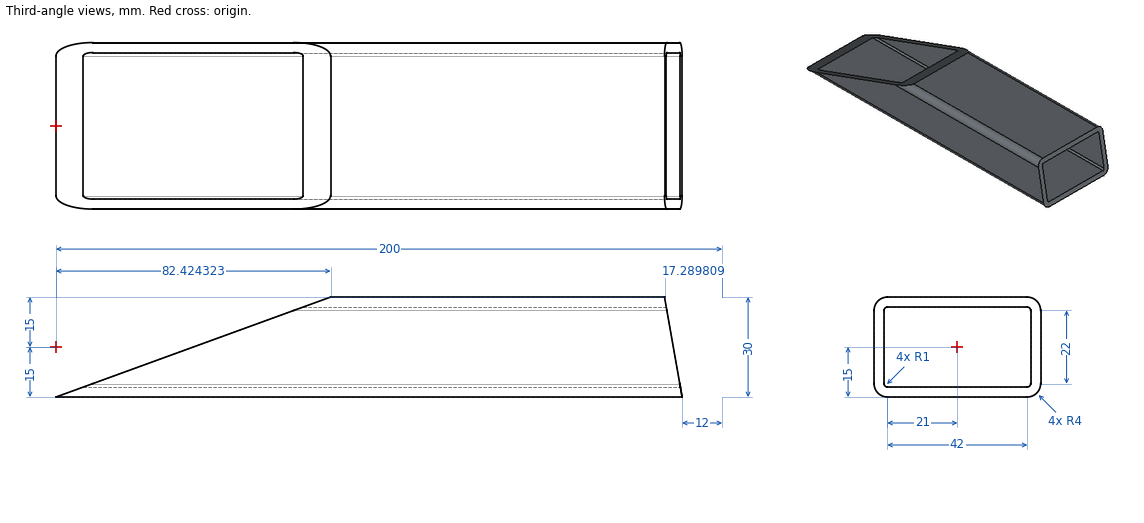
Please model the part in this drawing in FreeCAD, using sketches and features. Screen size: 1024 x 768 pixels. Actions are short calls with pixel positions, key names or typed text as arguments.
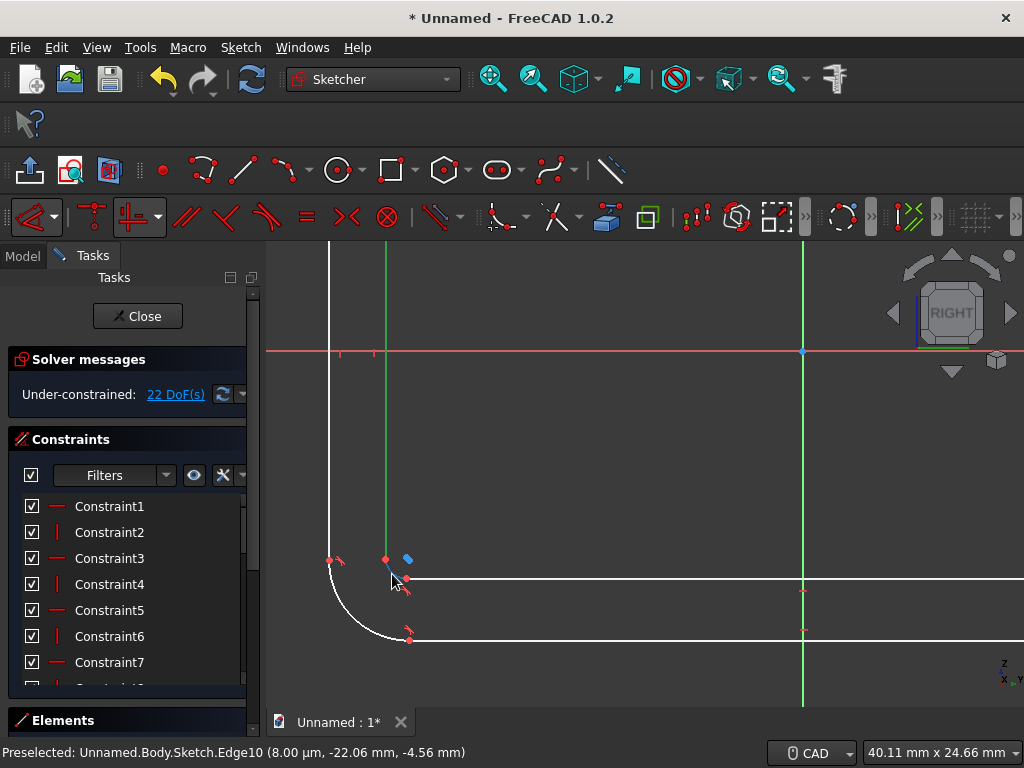
click(393, 573)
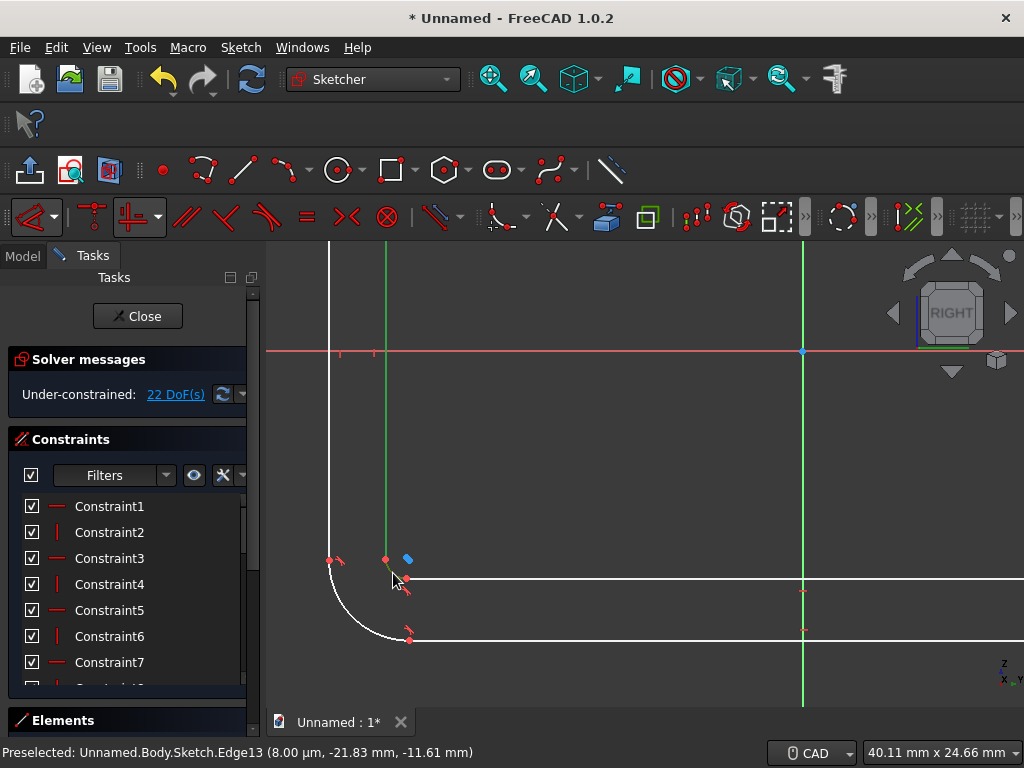
click(268, 218)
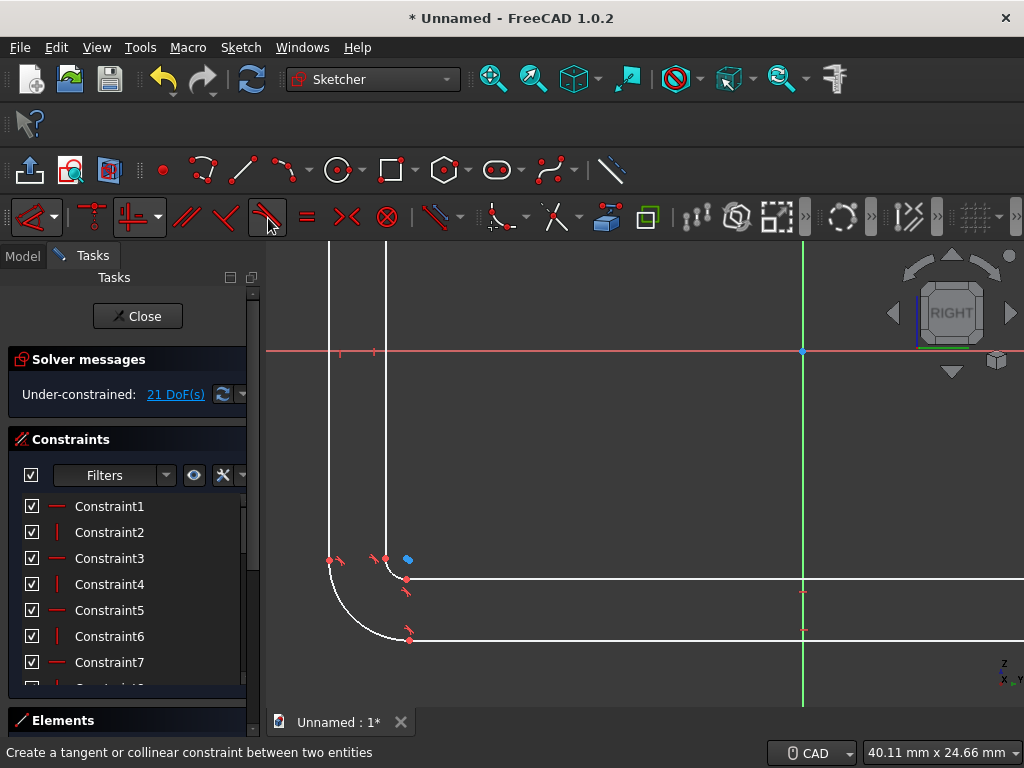
click(386, 434)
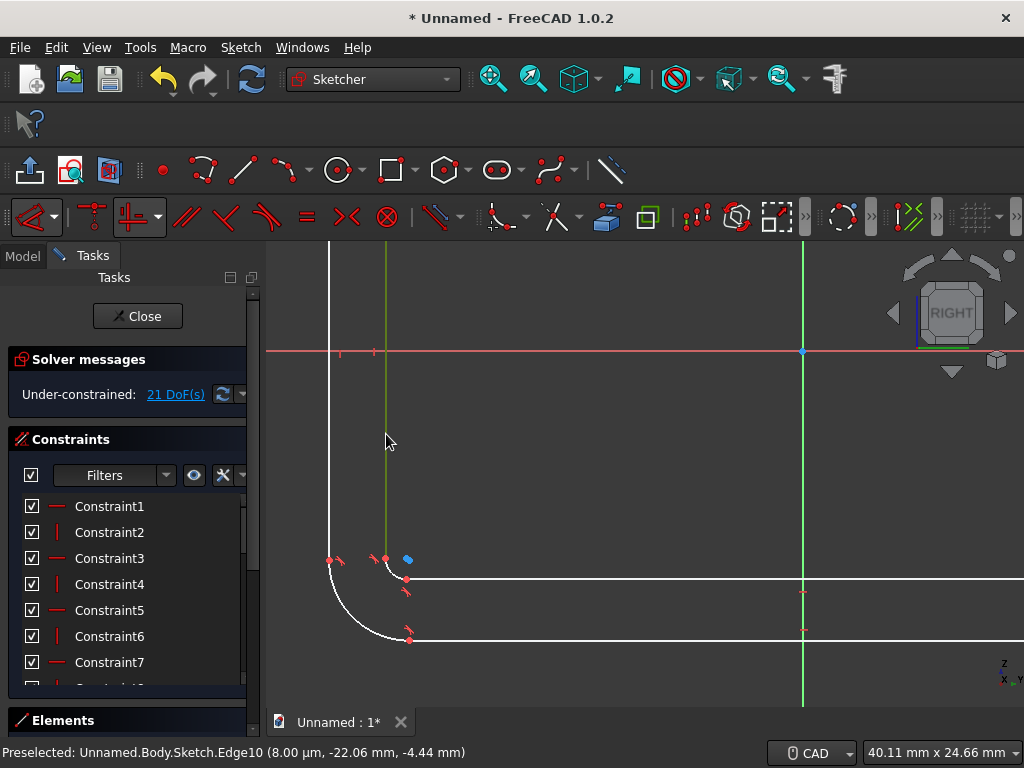
scroll(392, 574, down, 4)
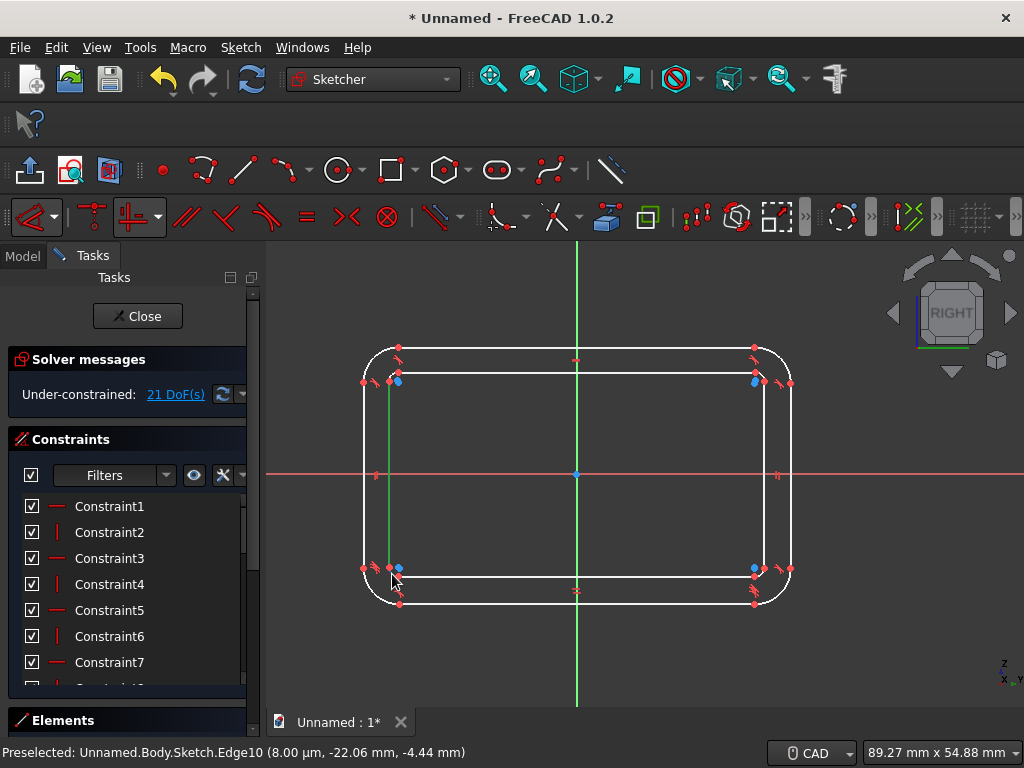
scroll(394, 373, up, 7)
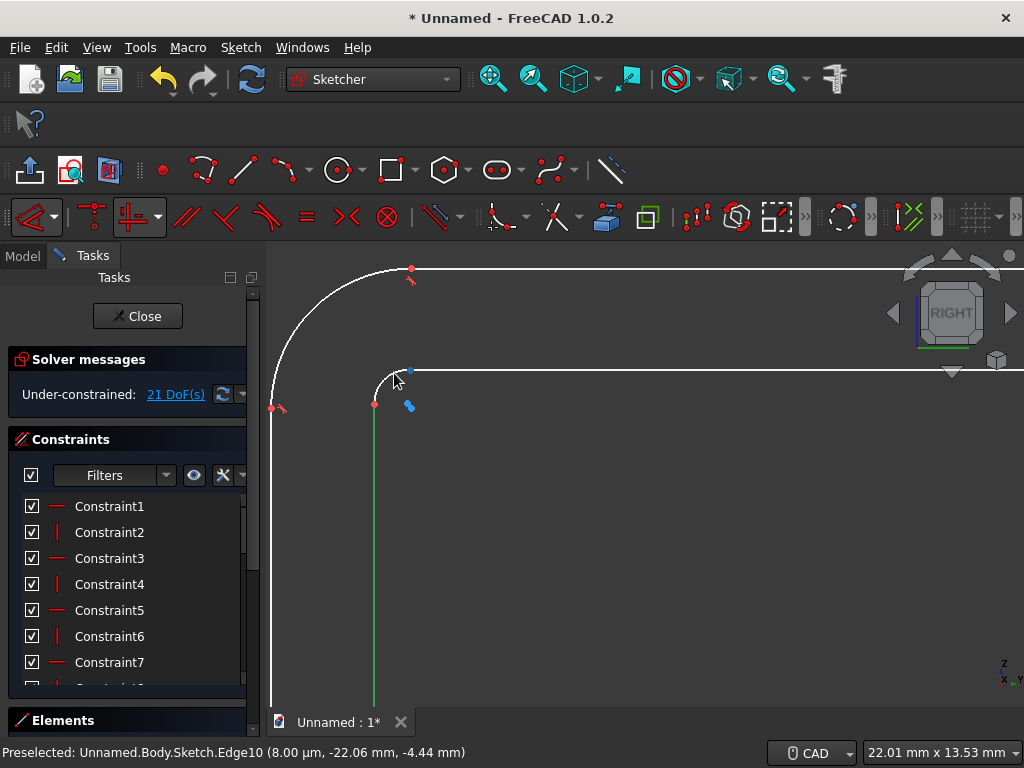
click(394, 373)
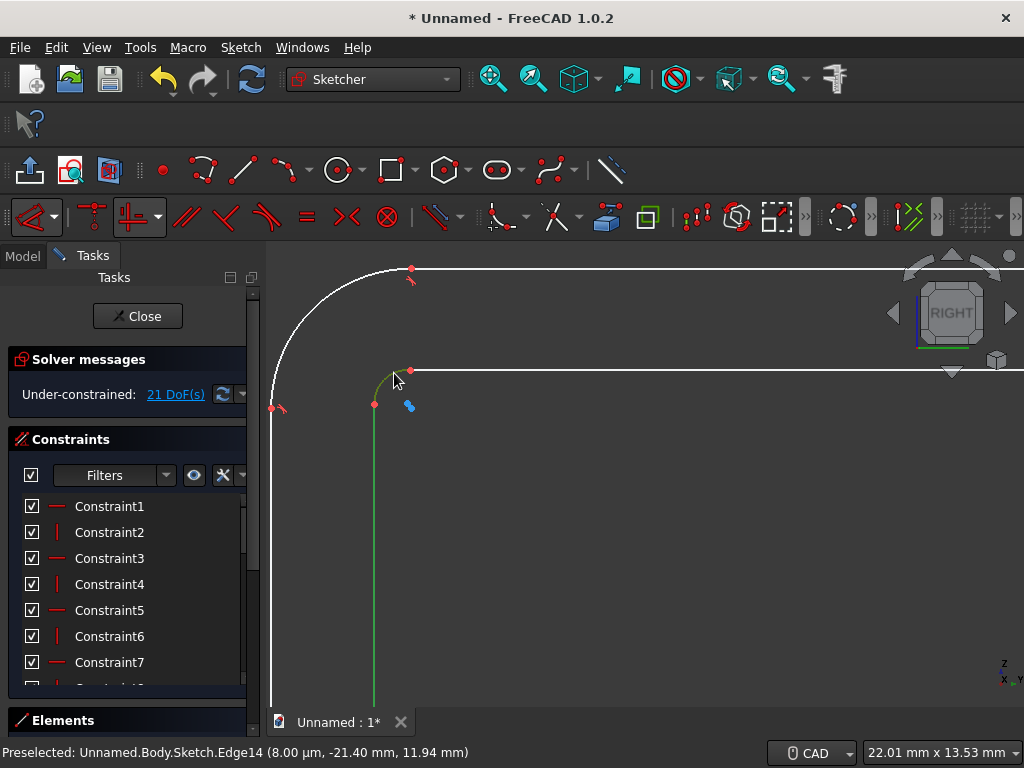
click(268, 218)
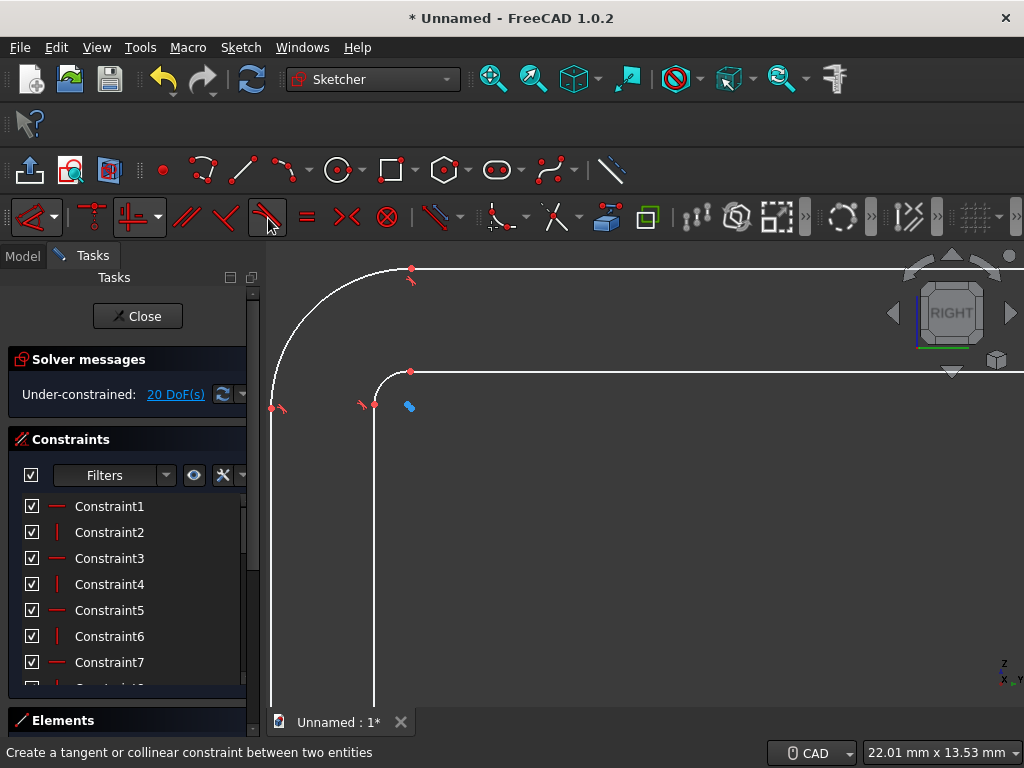
scroll(394, 373, down, 7)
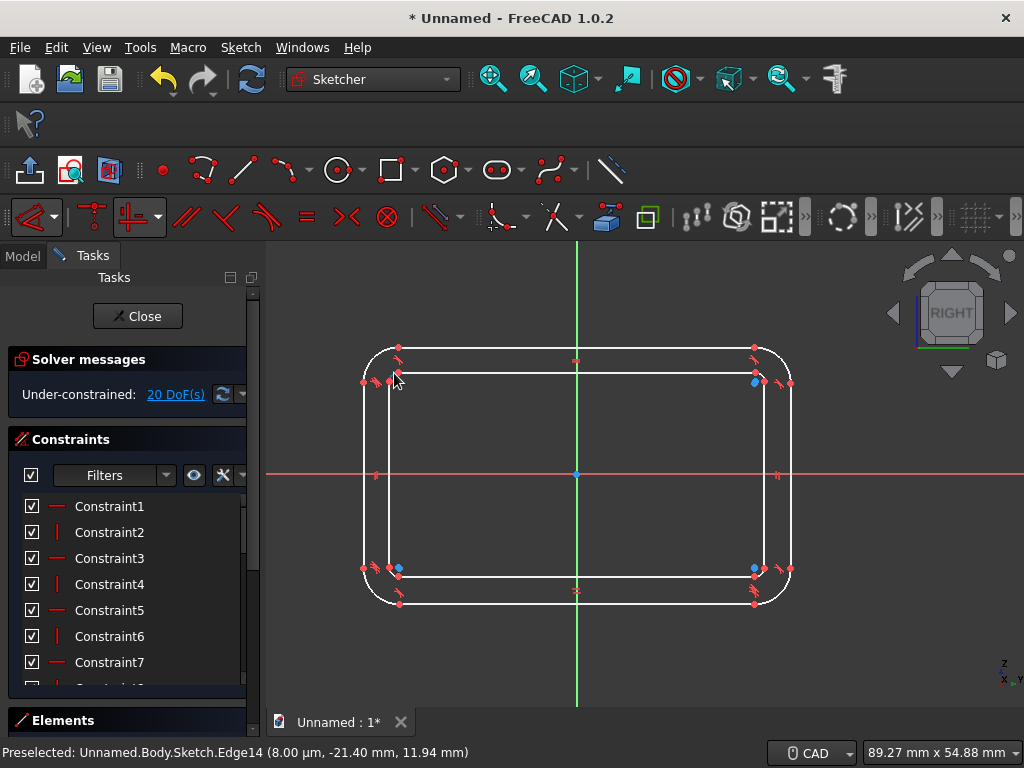
click(505, 373)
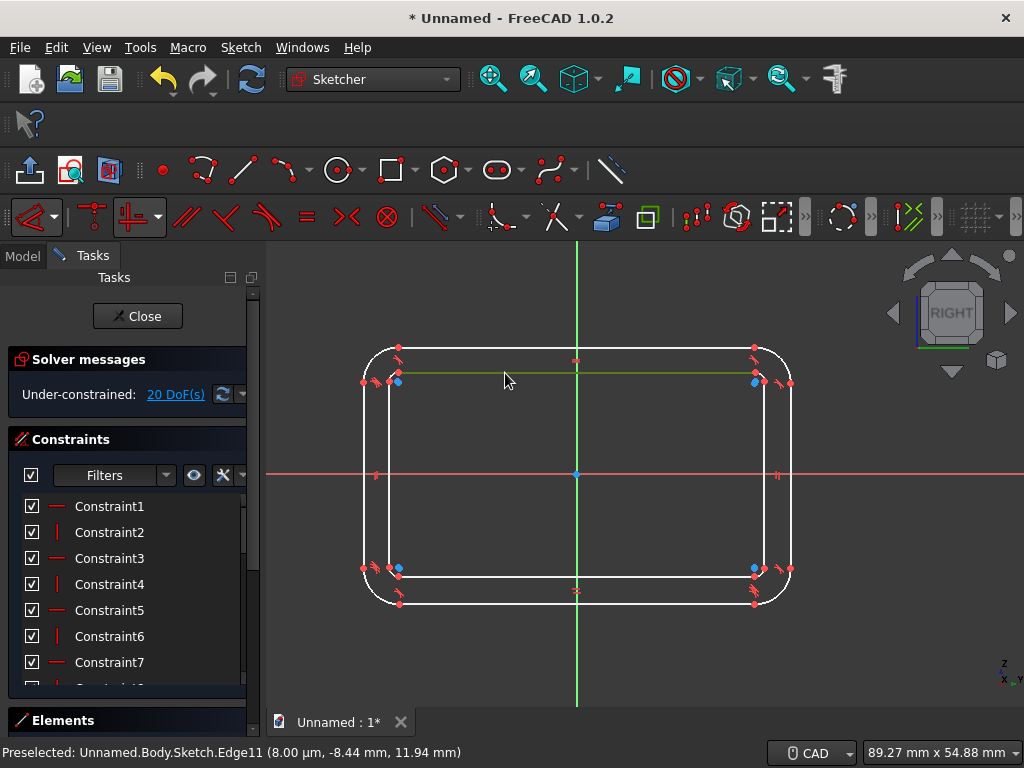
scroll(392, 375, up, 4)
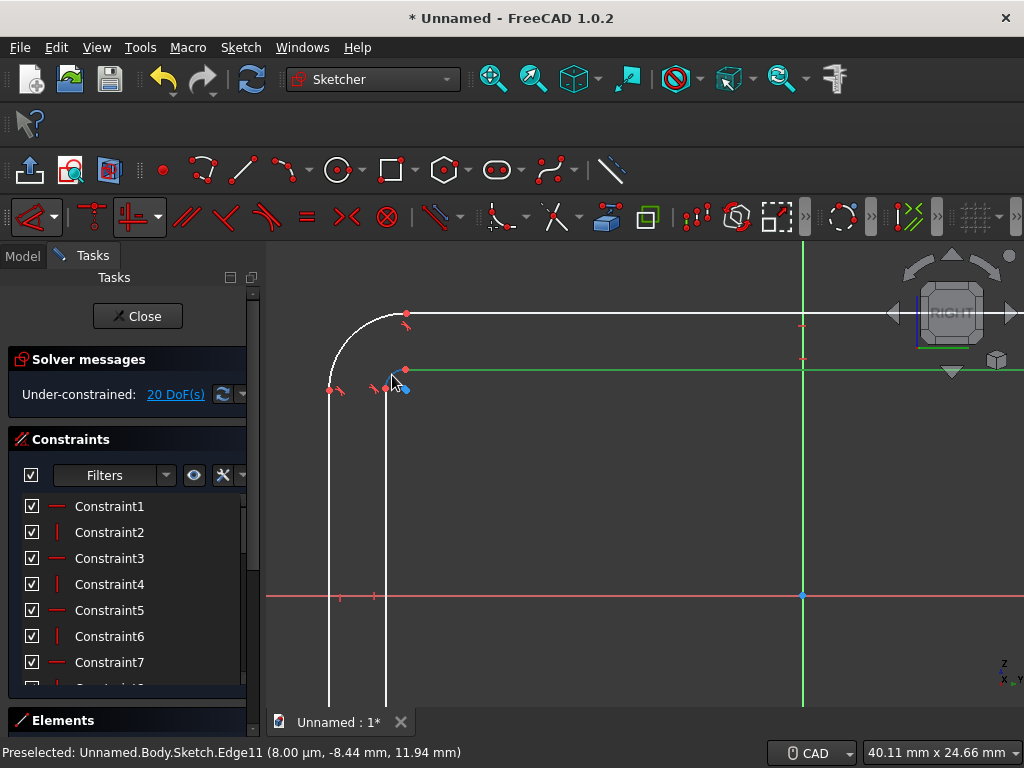
click(392, 375)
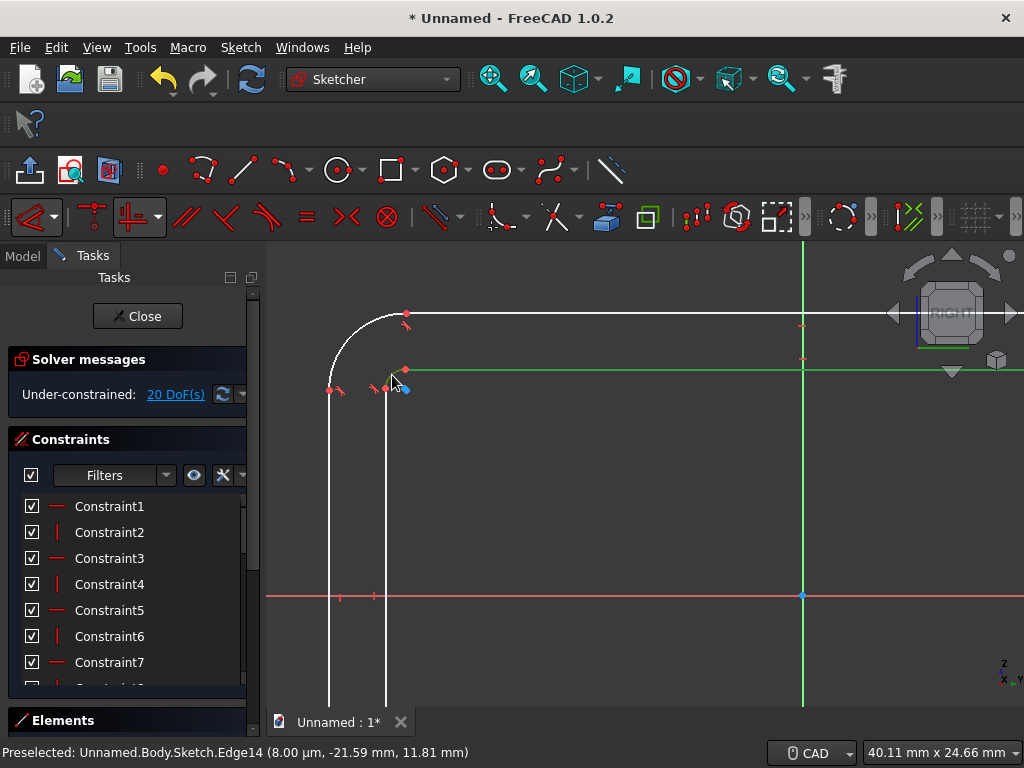
click(268, 218)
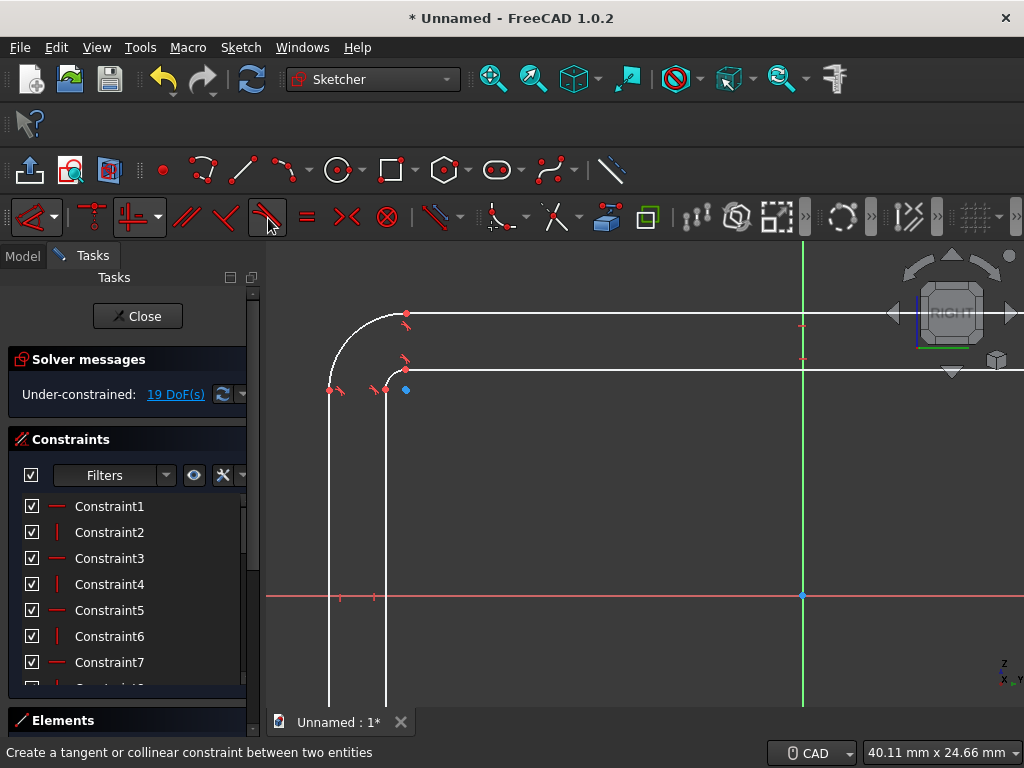
click(644, 370)